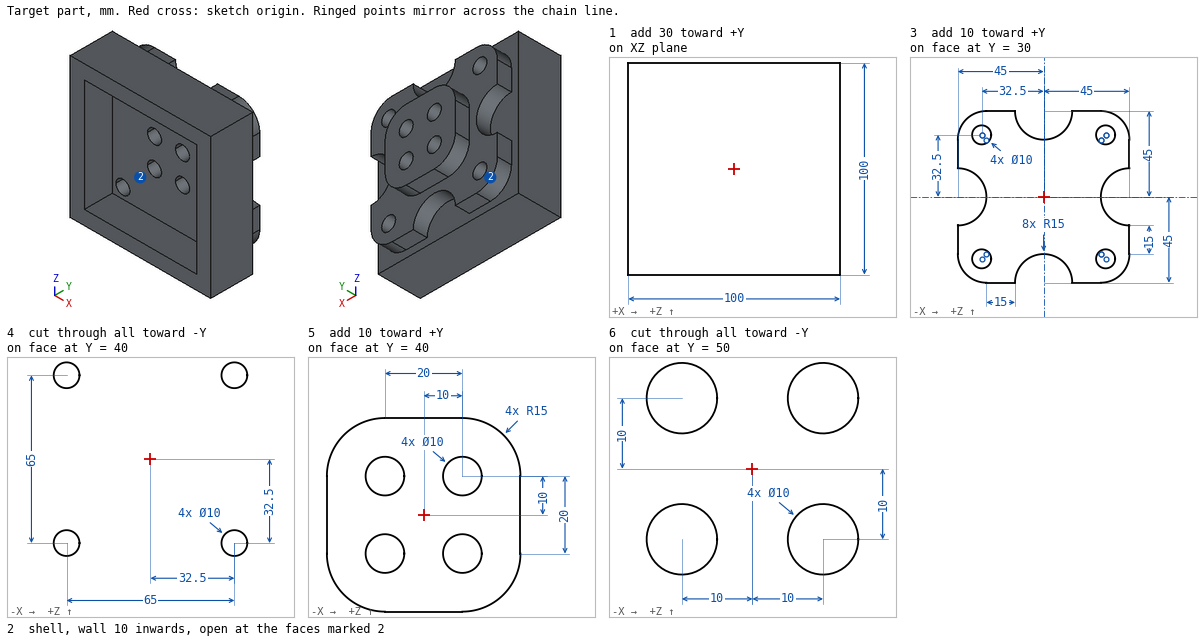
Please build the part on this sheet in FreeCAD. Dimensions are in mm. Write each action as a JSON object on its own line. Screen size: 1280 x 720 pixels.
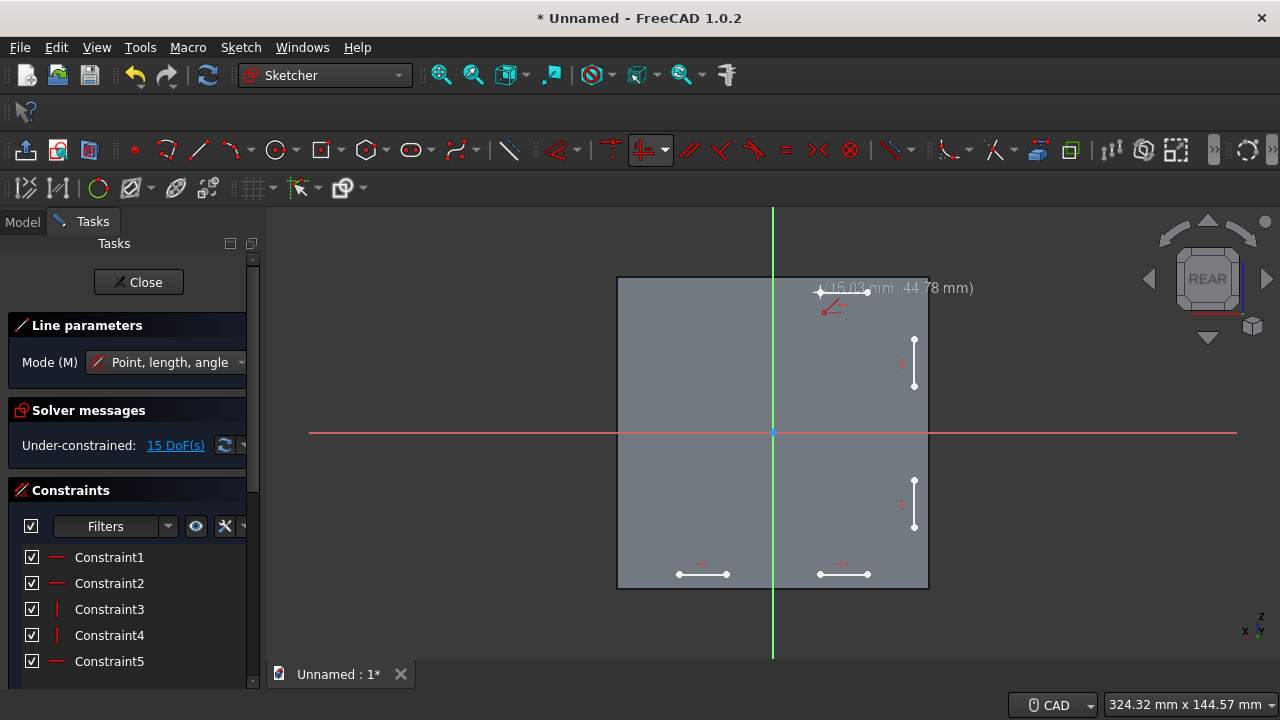
{"action": "left_click", "coordinate": [726, 292]}
{"action": "left_click", "coordinate": [679, 292]}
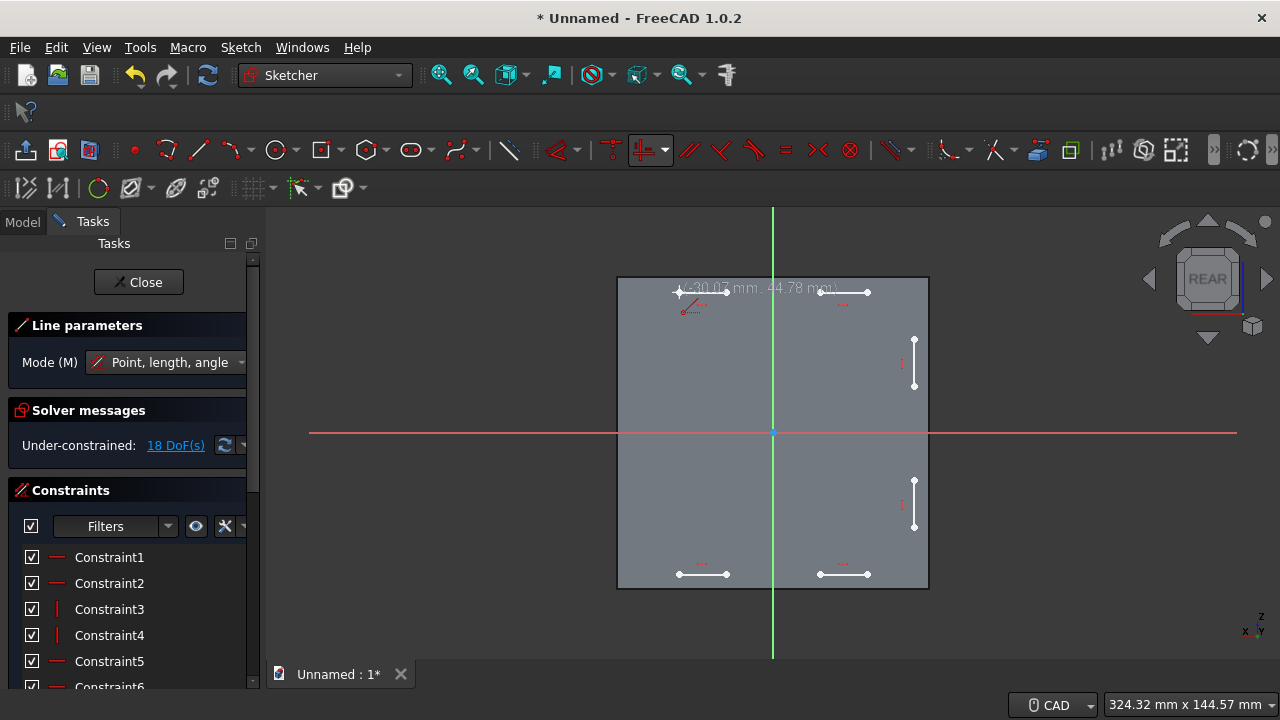
{"action": "left_click", "coordinate": [632, 339]}
{"action": "left_click", "coordinate": [632, 386]}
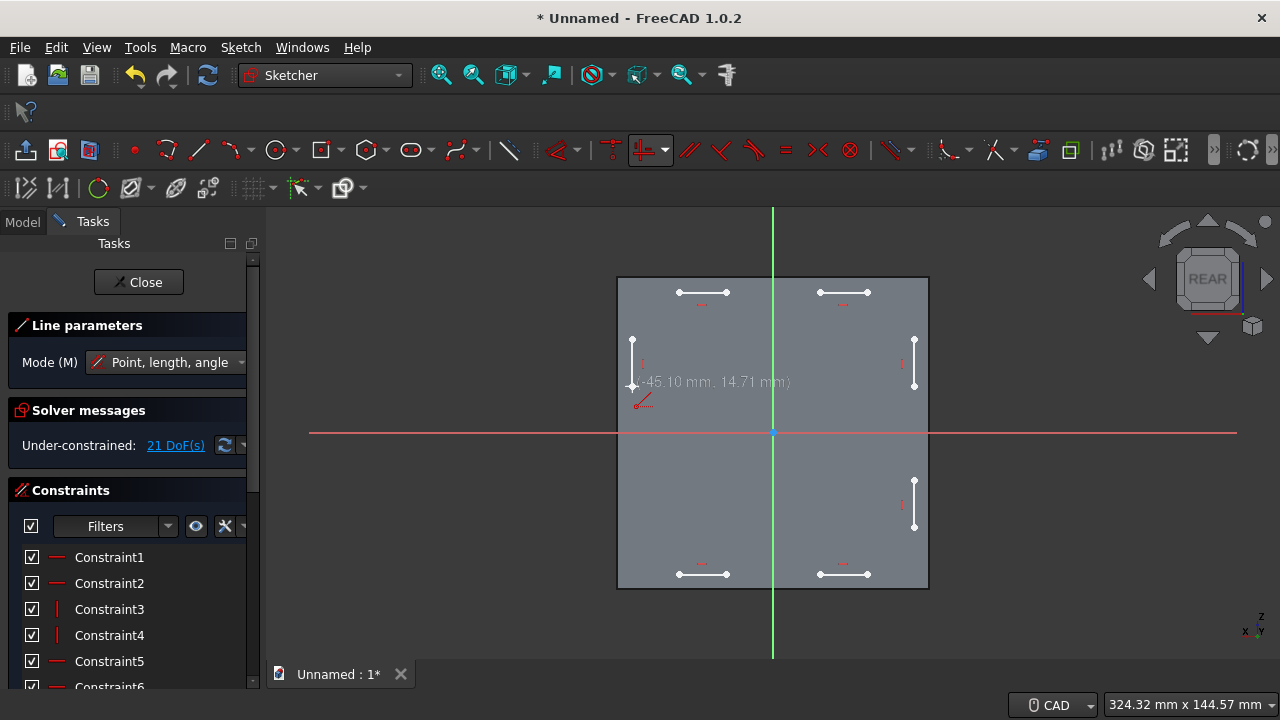
{"action": "left_click", "coordinate": [632, 480]}
{"action": "left_click", "coordinate": [632, 527]}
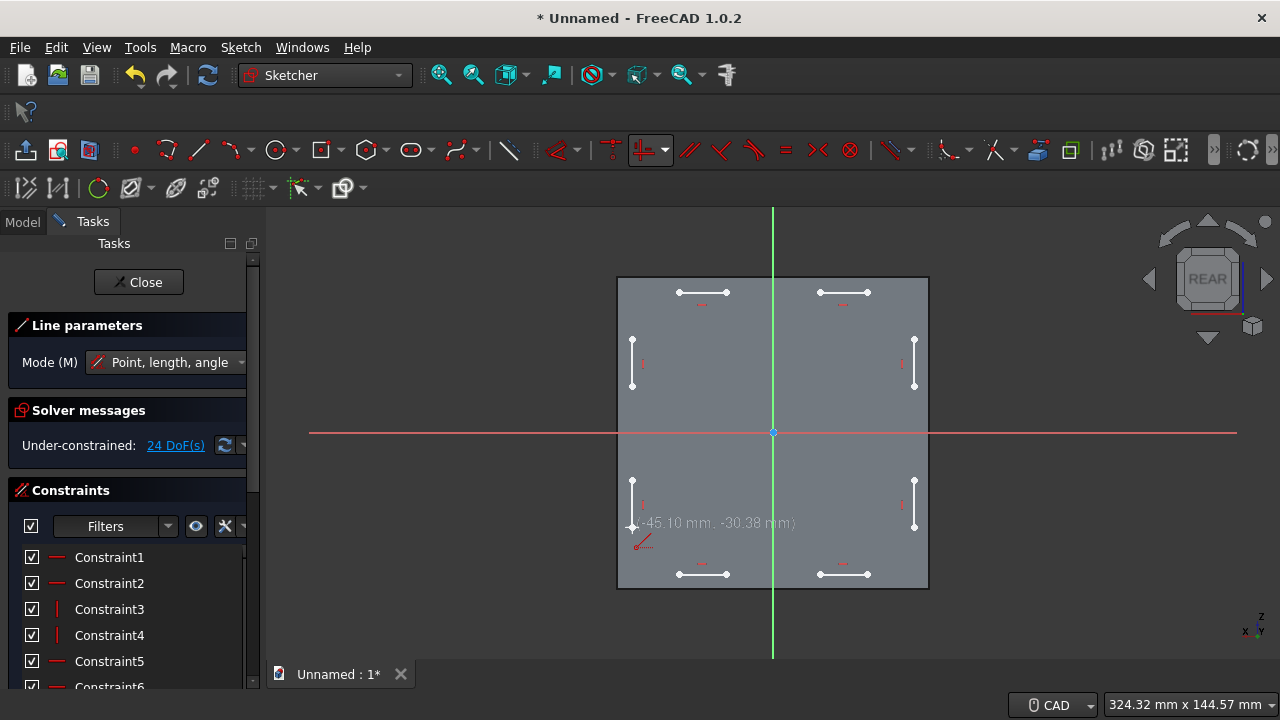
{"action": "left_click", "coordinate": [232, 150]}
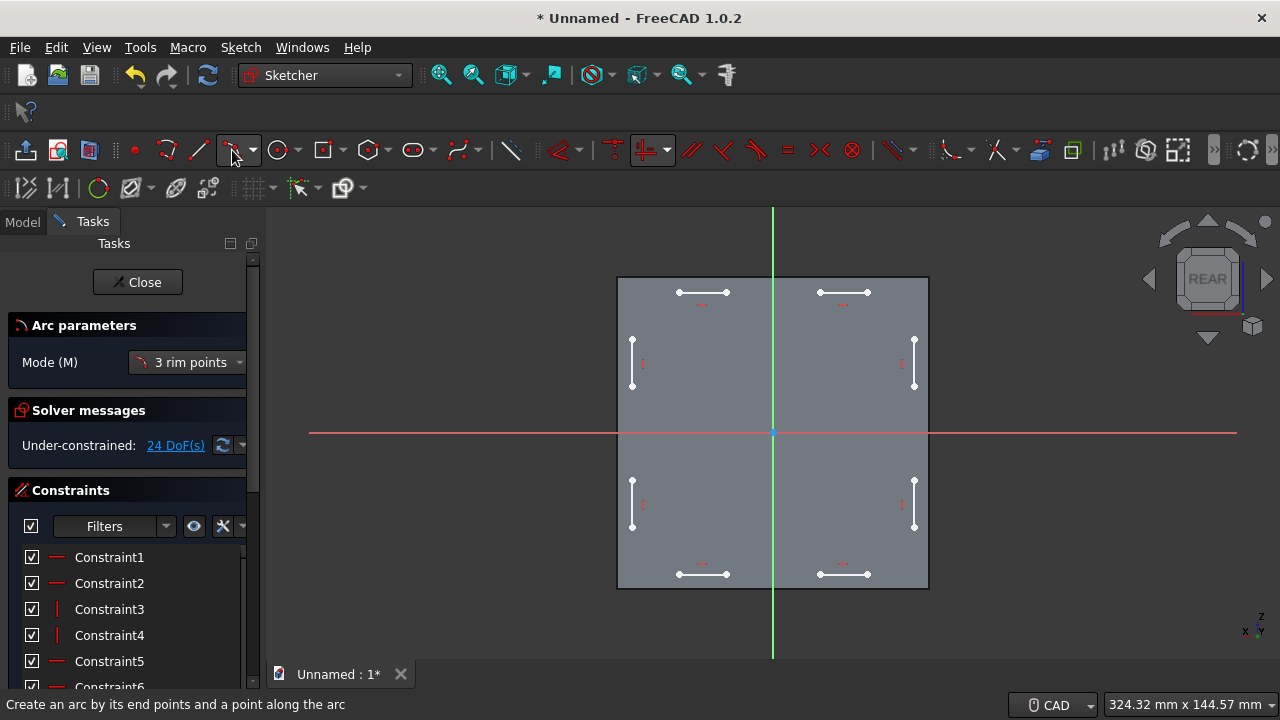
{"action": "left_click", "coordinate": [726, 575]}
{"action": "left_click", "coordinate": [820, 575]}
{"action": "left_click", "coordinate": [787, 529]}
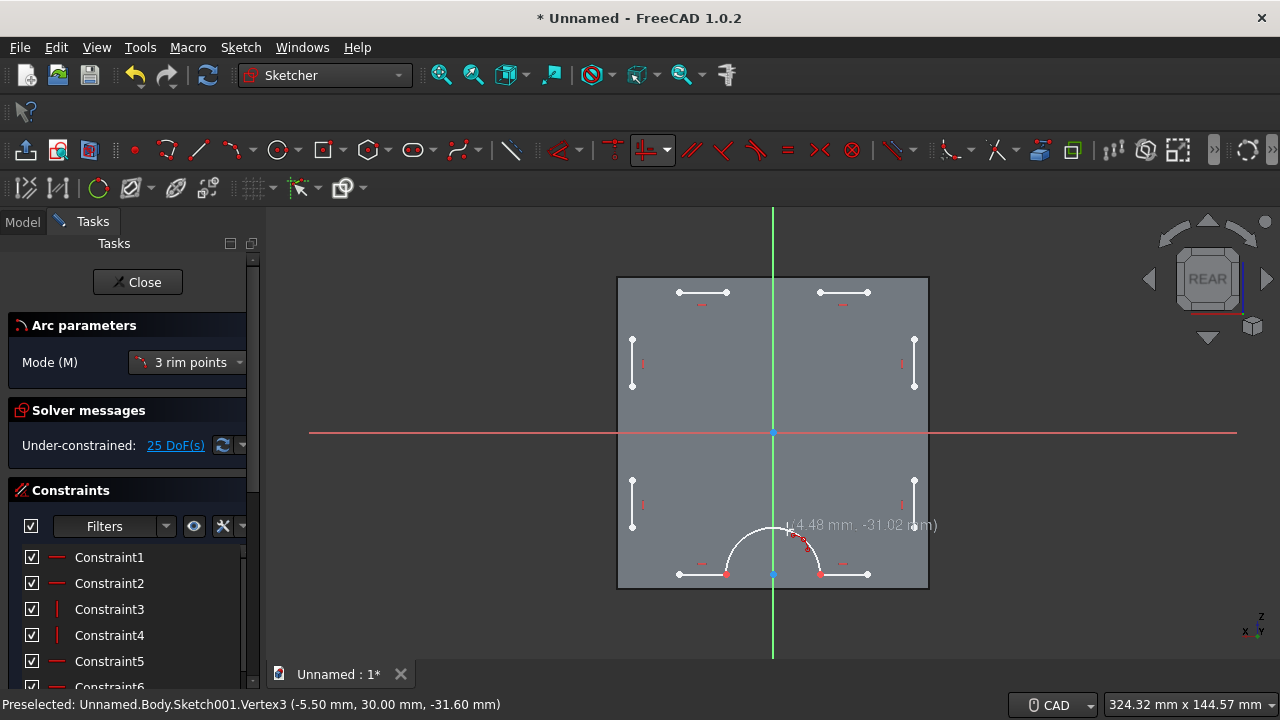
{"action": "left_click", "coordinate": [867, 575]}
{"action": "left_click", "coordinate": [914, 528]}
{"action": "left_click", "coordinate": [900, 560]}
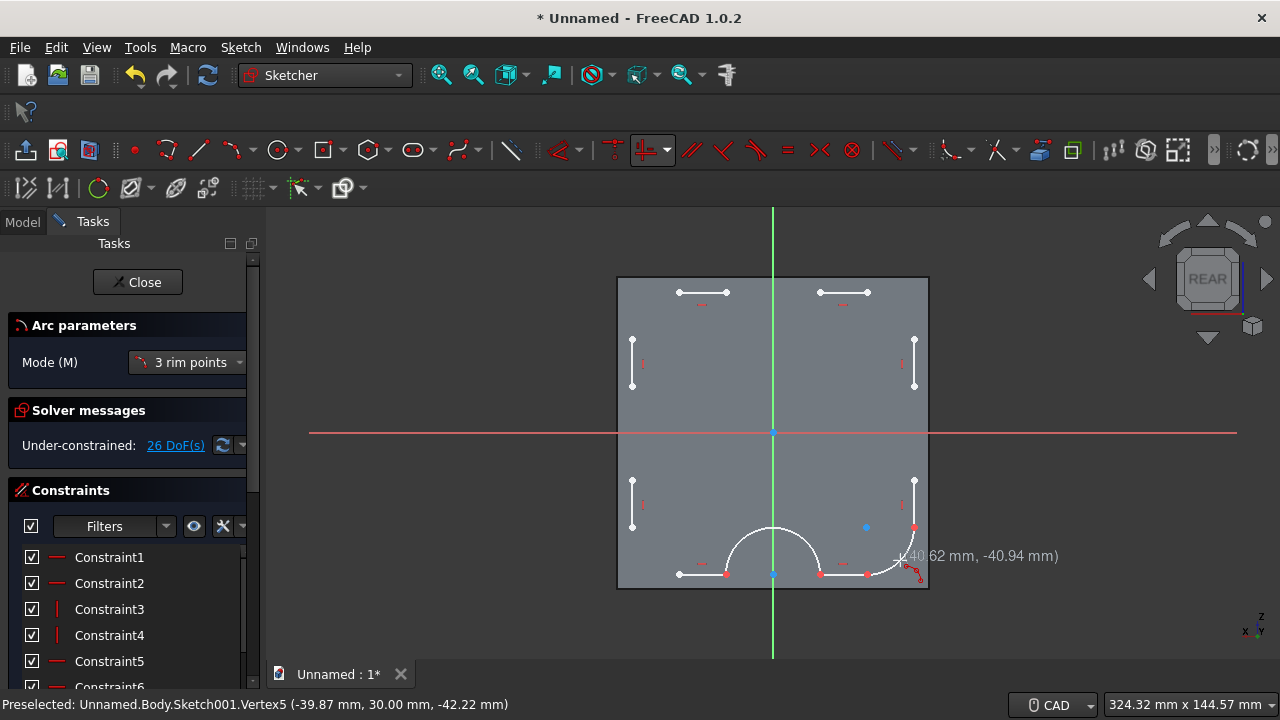
{"action": "left_click", "coordinate": [914, 481]}
{"action": "left_click", "coordinate": [914, 387]}
{"action": "left_click", "coordinate": [869, 419]}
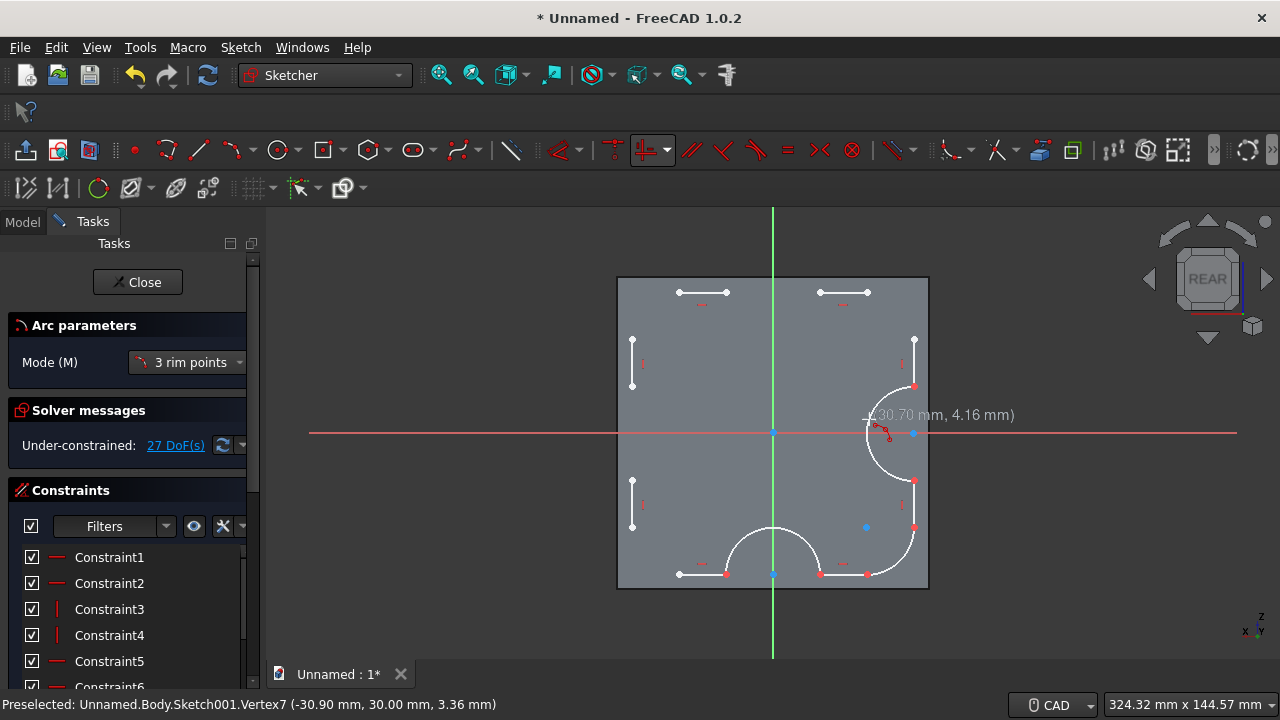
{"action": "left_click", "coordinate": [914, 340]}
{"action": "left_click", "coordinate": [867, 293]}
{"action": "left_click", "coordinate": [900, 306]}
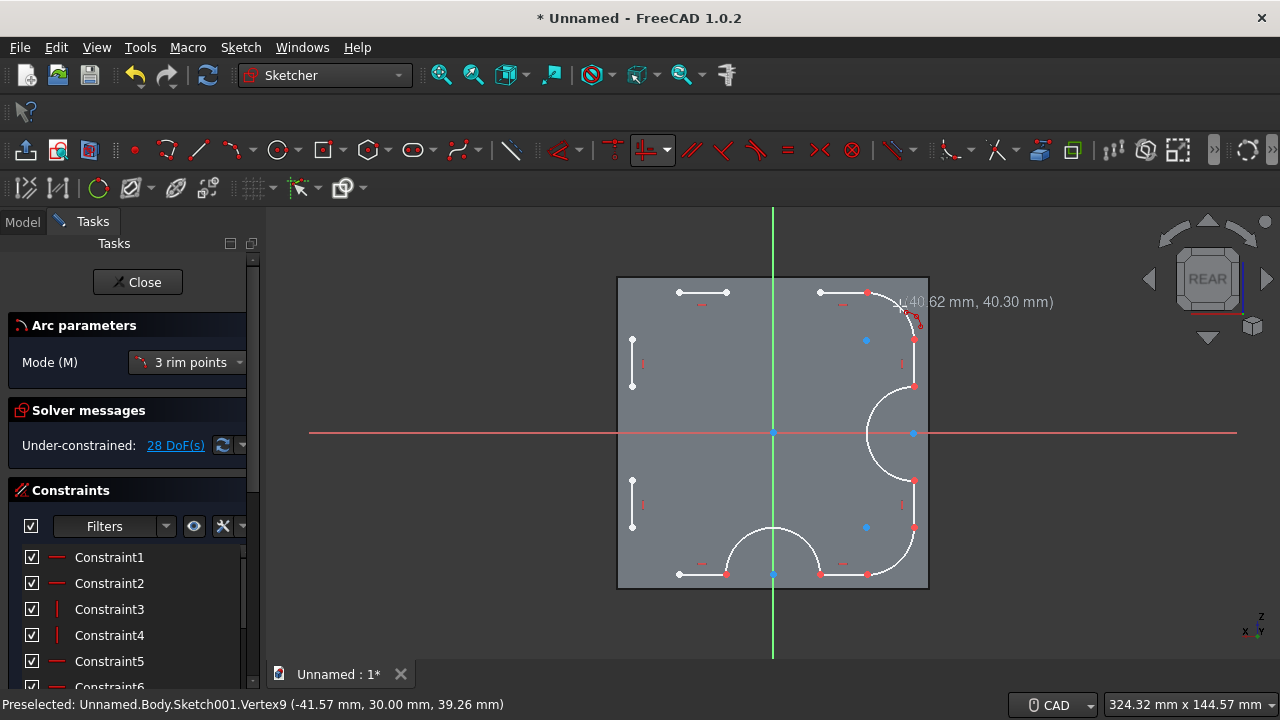
{"action": "left_click", "coordinate": [820, 293]}
{"action": "left_click", "coordinate": [726, 293]}
{"action": "left_click", "coordinate": [759, 337]}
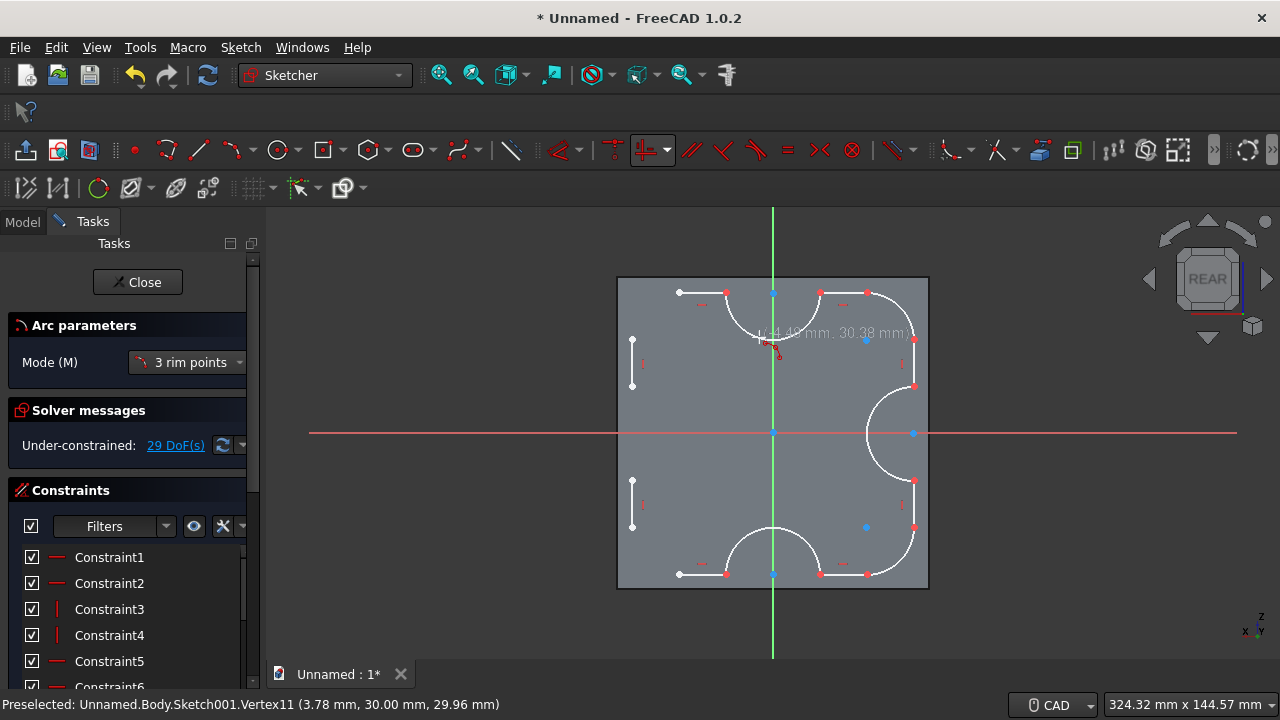
{"action": "left_click", "coordinate": [679, 293]}
{"action": "left_click", "coordinate": [632, 340]}
{"action": "left_click", "coordinate": [646, 306]}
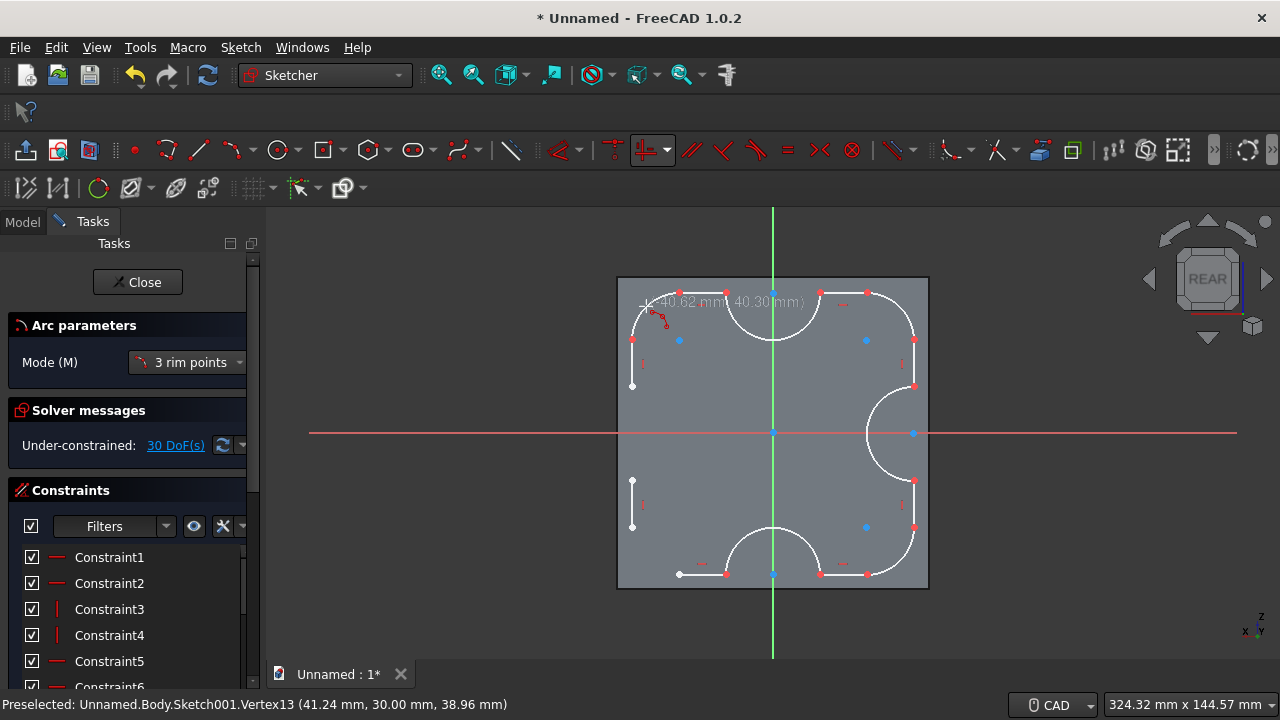
{"action": "left_click", "coordinate": [632, 387]}
{"action": "left_click", "coordinate": [632, 481]}
{"action": "left_click", "coordinate": [677, 447]}